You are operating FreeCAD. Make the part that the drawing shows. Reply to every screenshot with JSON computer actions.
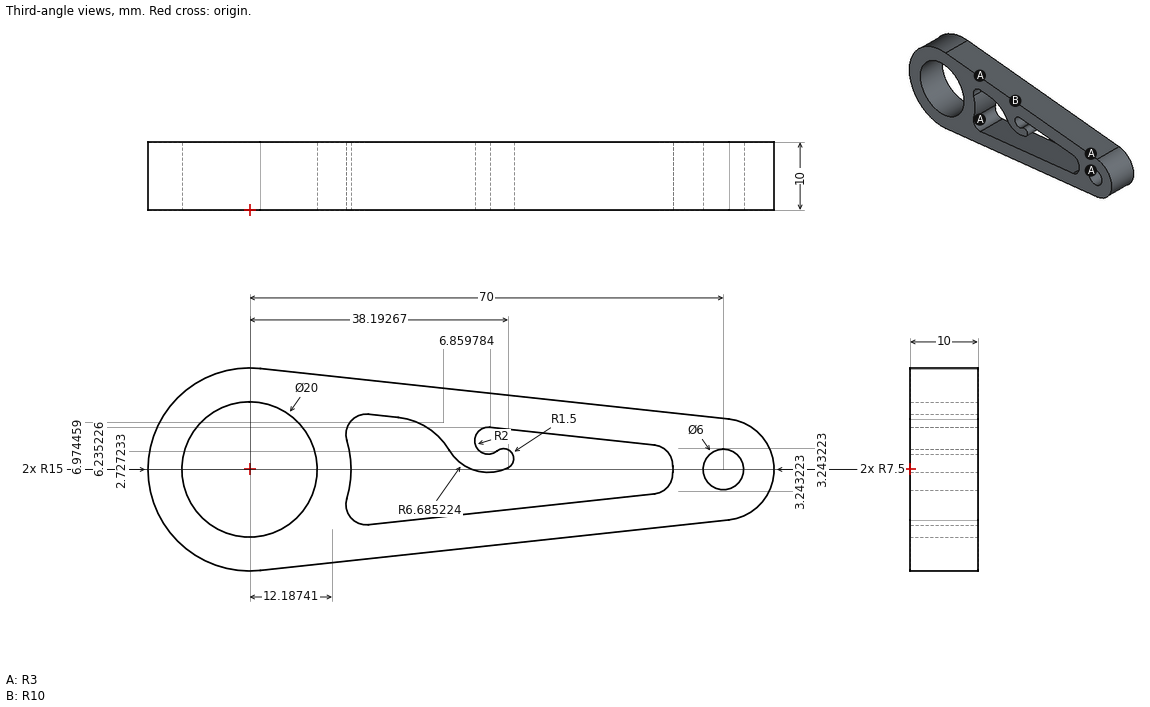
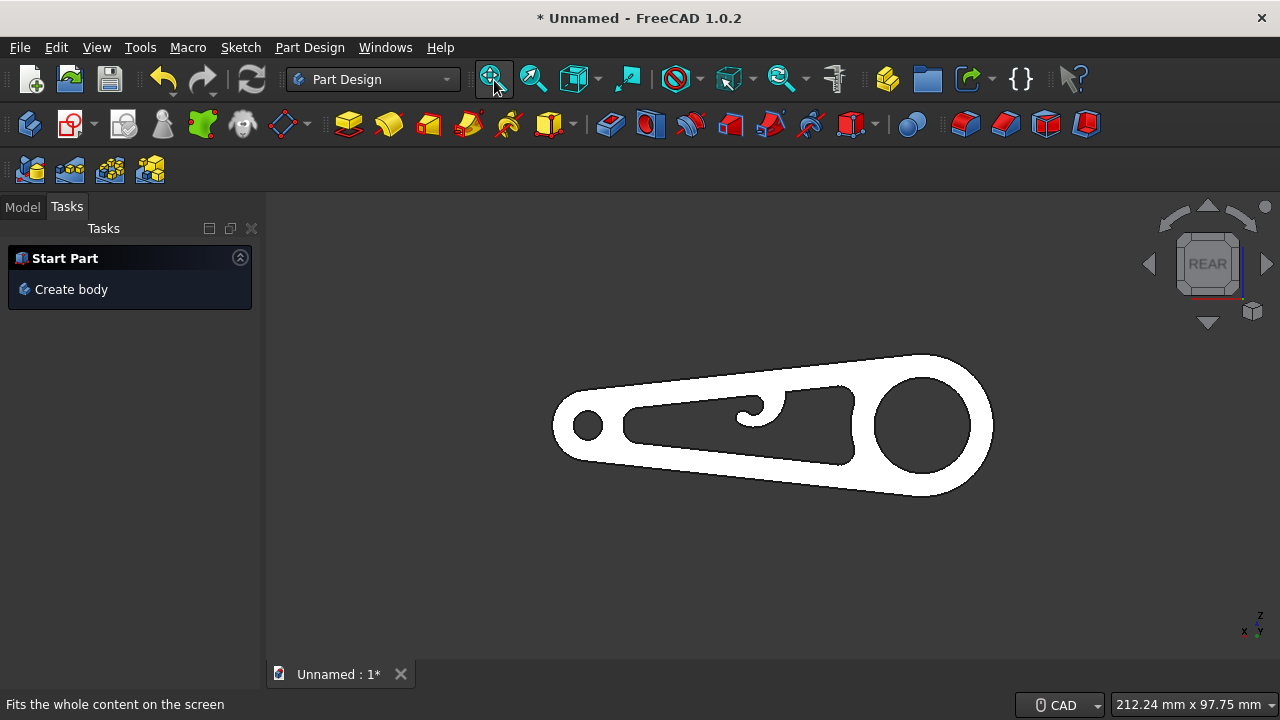
{"action": "left_click", "coordinate": [494, 80]}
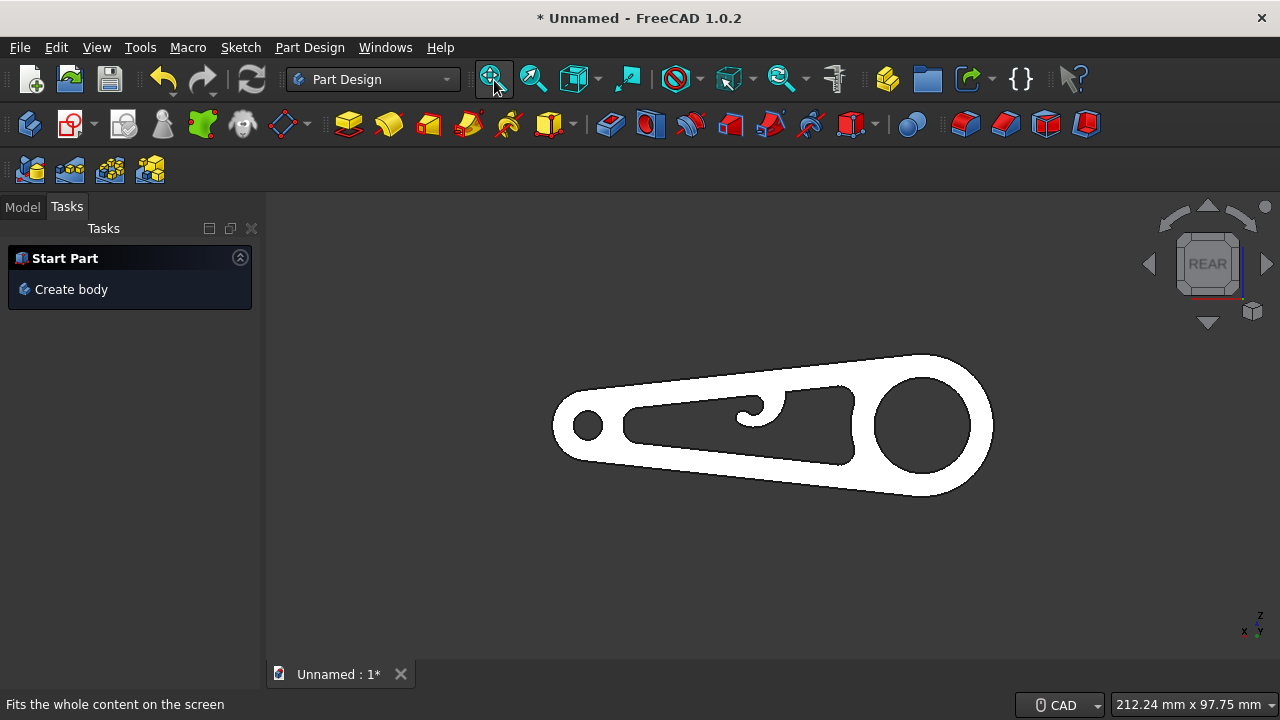
{"action": "key", "text": "6"}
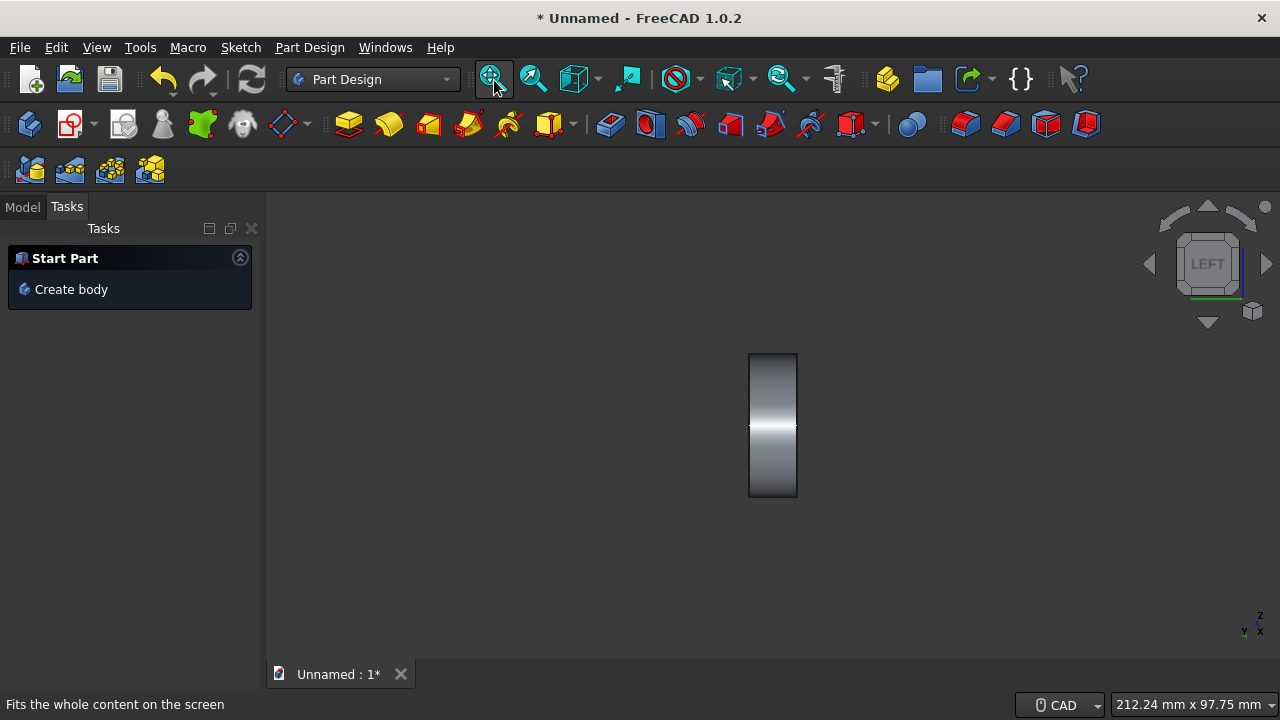
{"action": "left_click", "coordinate": [494, 80]}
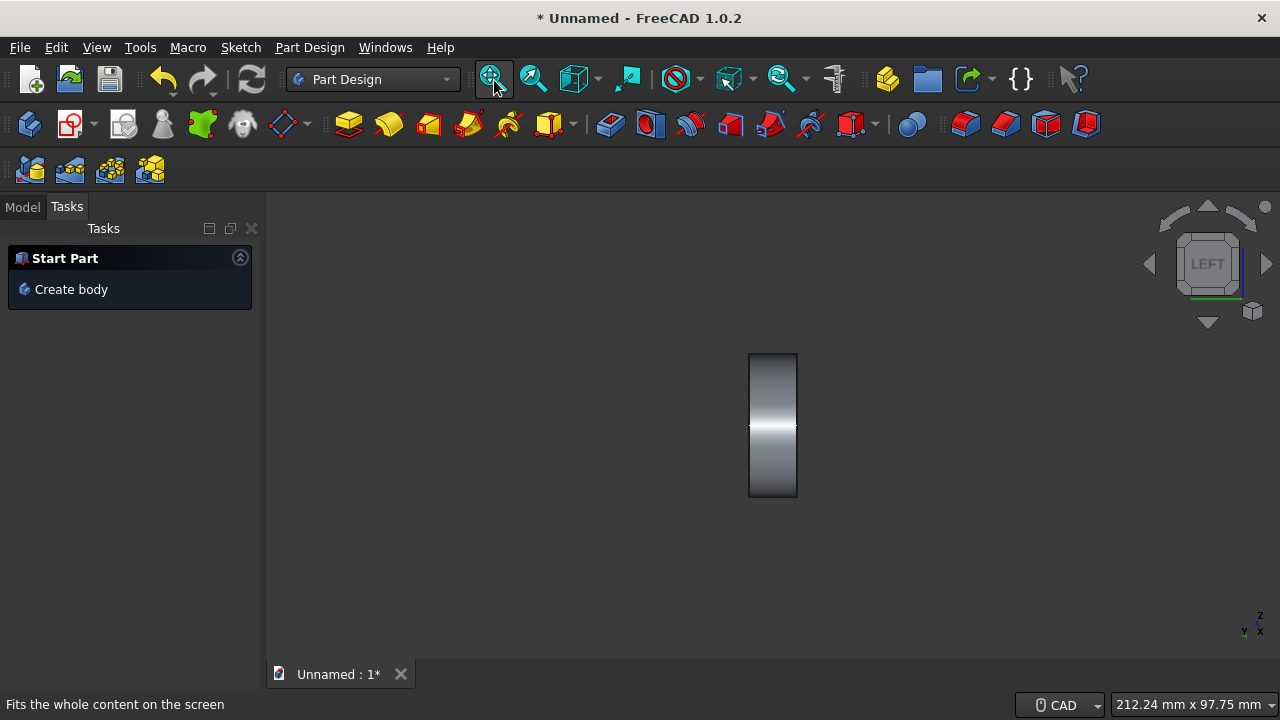
{"action": "key", "text": "v 3"}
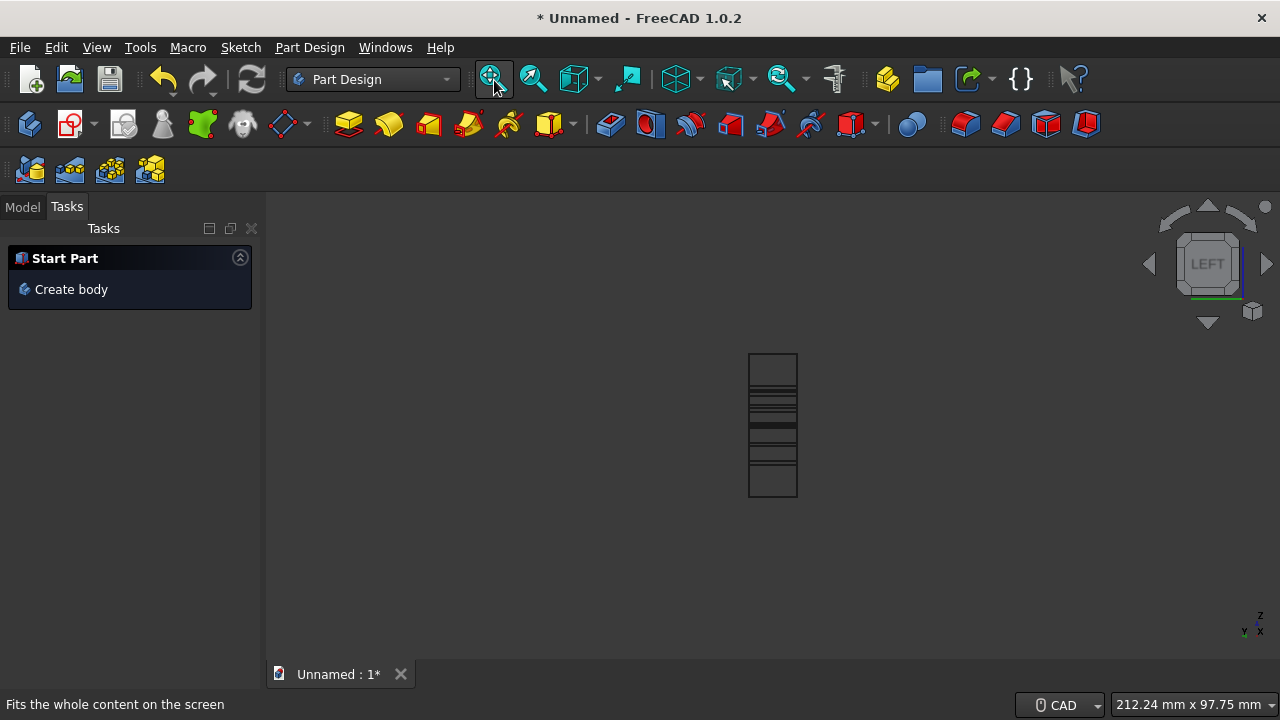
{"action": "key", "text": "0"}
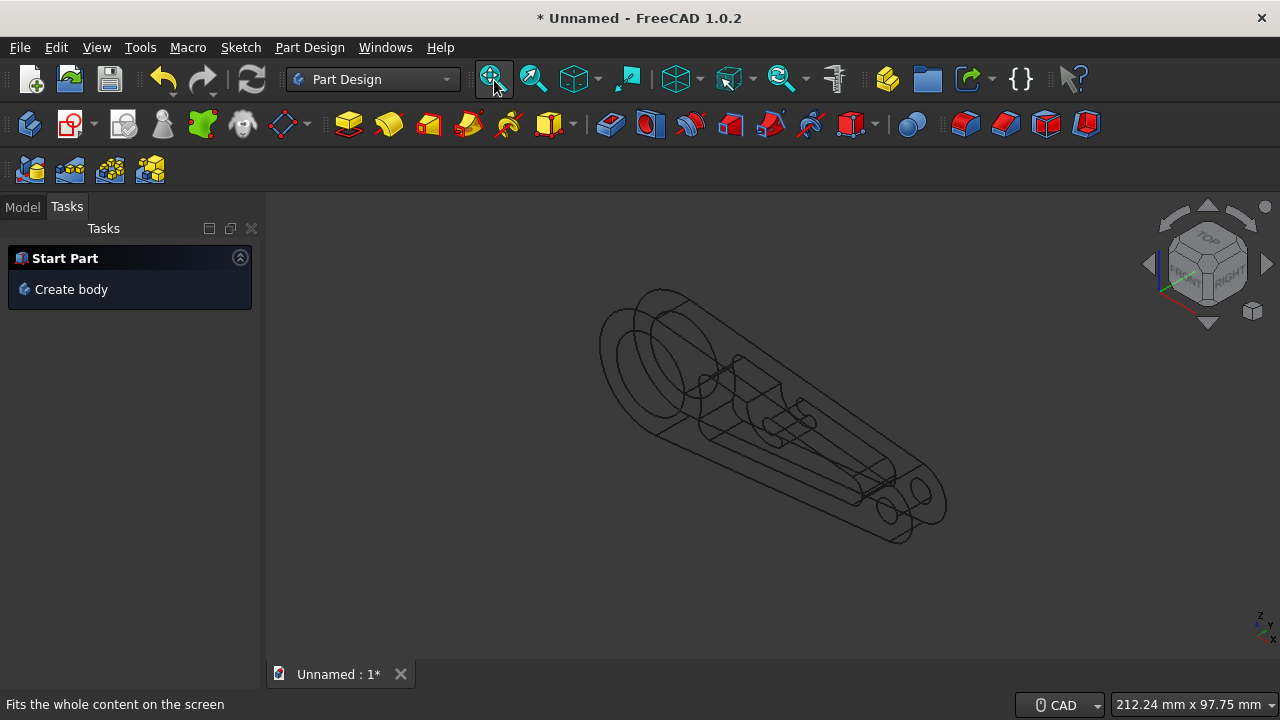
{"action": "left_click", "coordinate": [771, 388]}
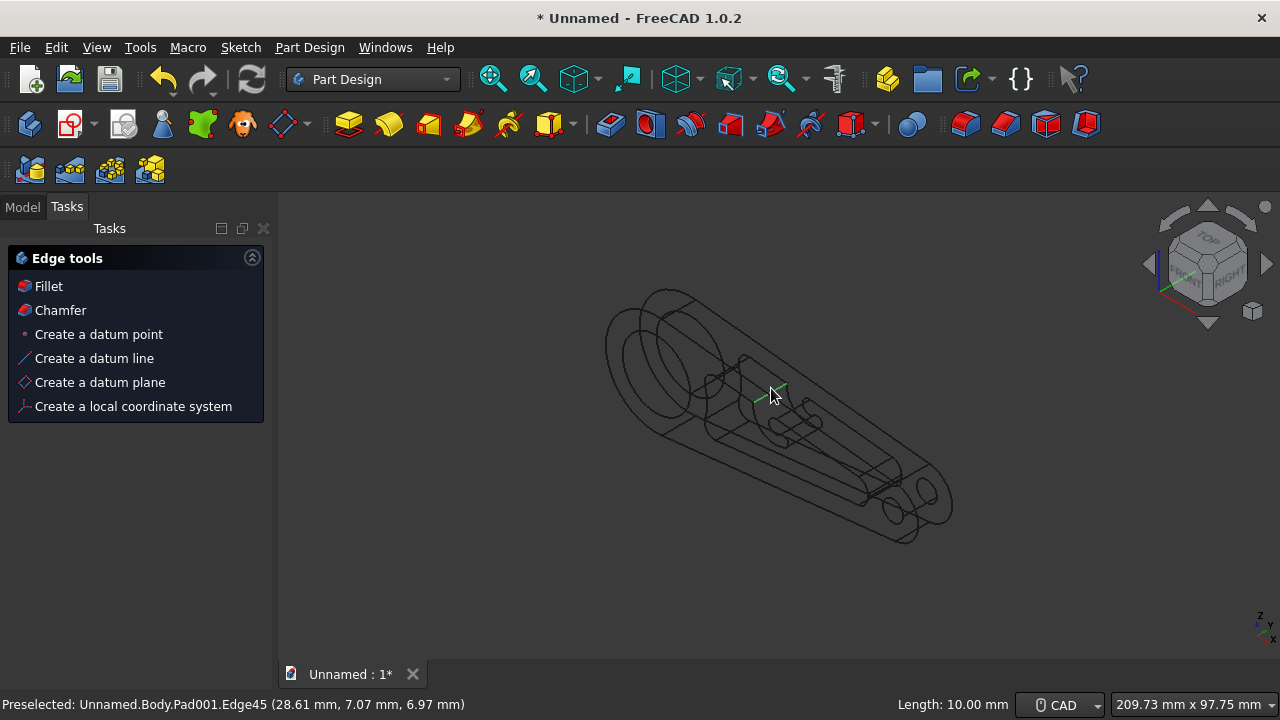
{"action": "key", "text": "v 1"}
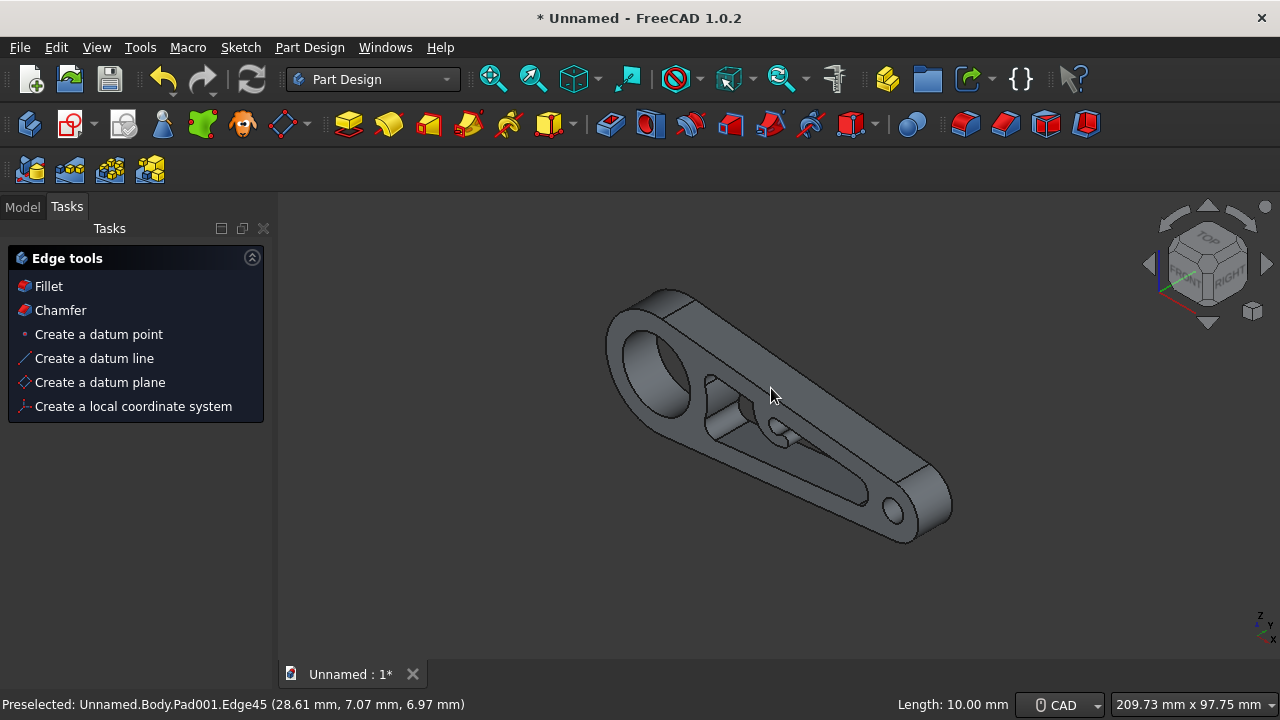
{"action": "left_click", "coordinate": [966, 124]}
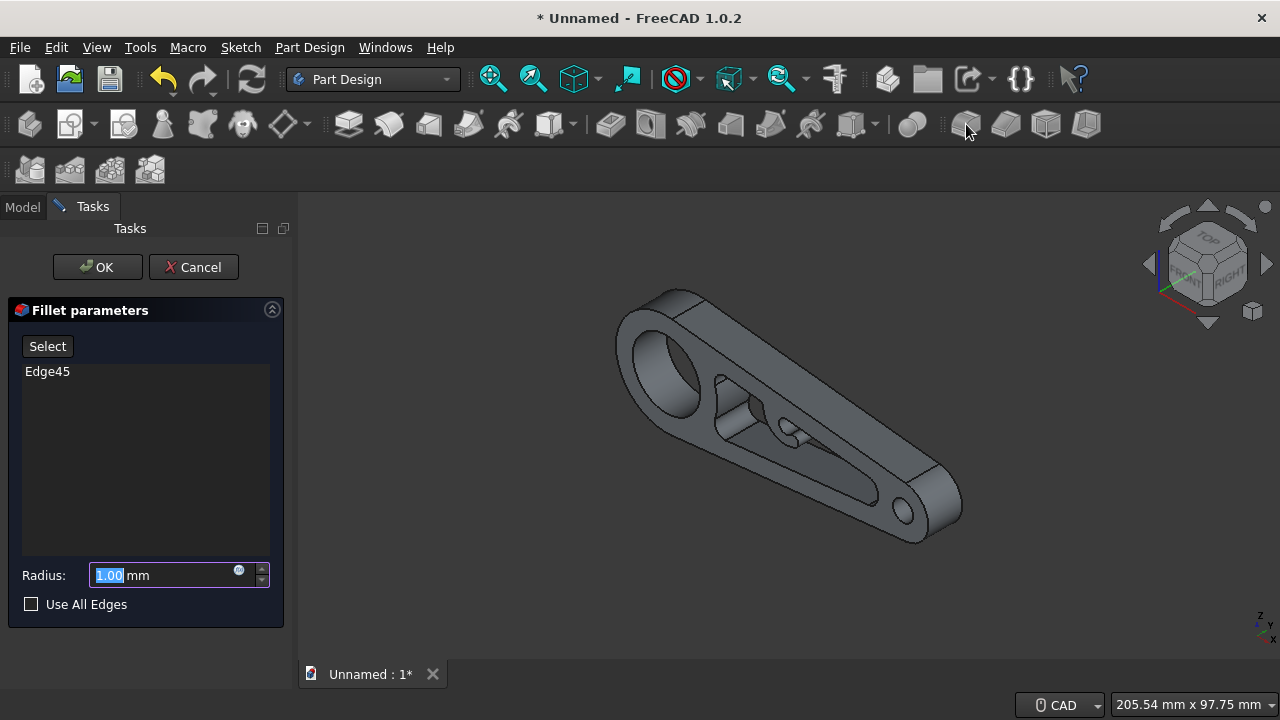
{"action": "type", "text": "10"}
{"action": "key", "text": "Tab"}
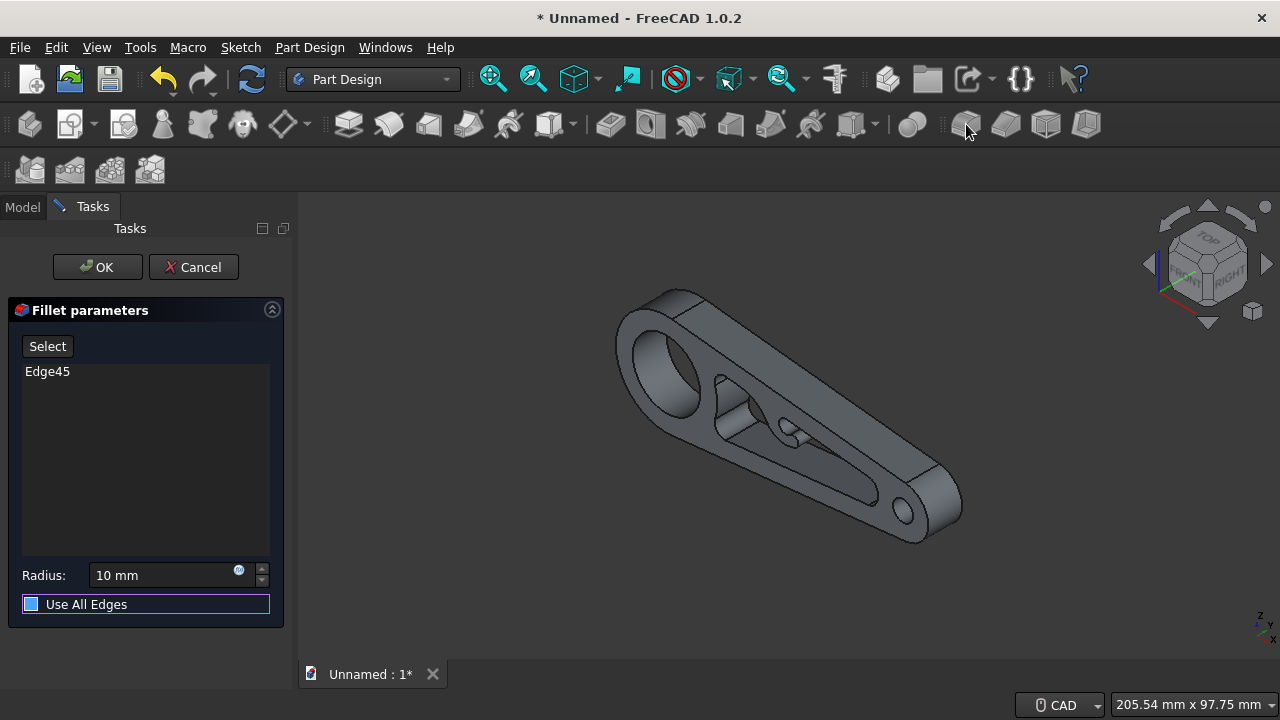
{"action": "left_click", "coordinate": [98, 267]}